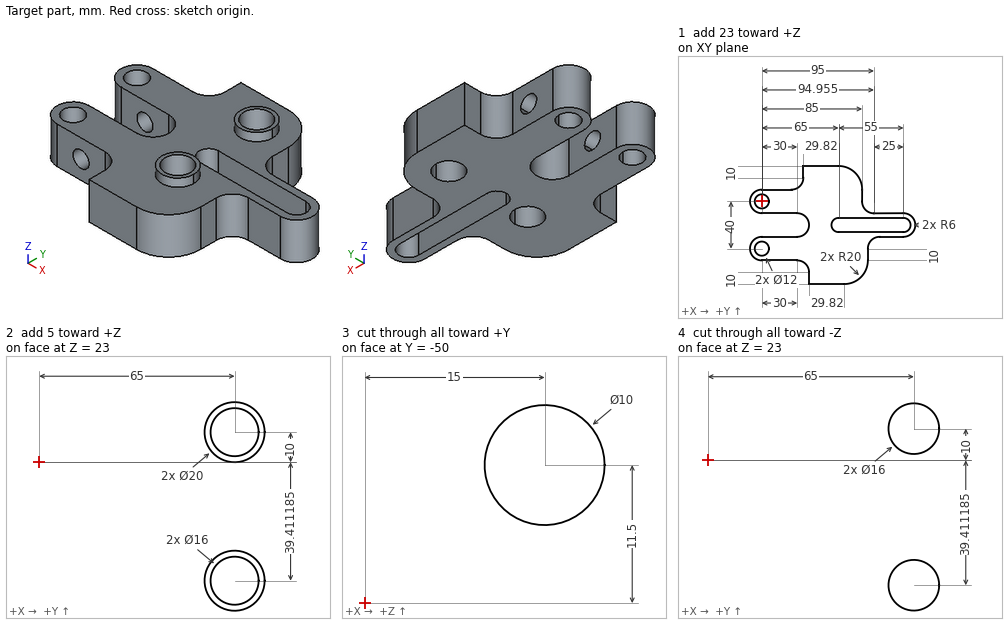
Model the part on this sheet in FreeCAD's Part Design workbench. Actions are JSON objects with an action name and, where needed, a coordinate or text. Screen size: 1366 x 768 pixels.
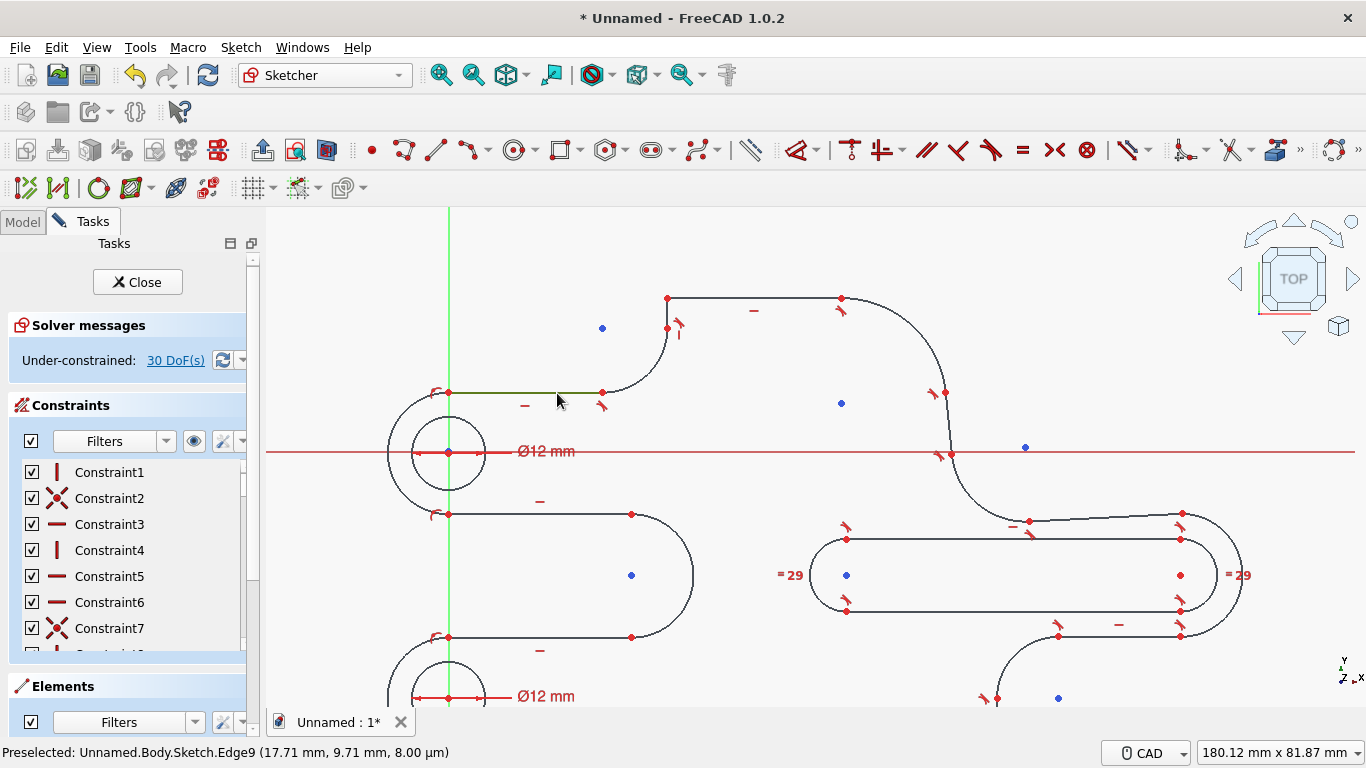
{"action": "left_click", "coordinate": [400, 418]}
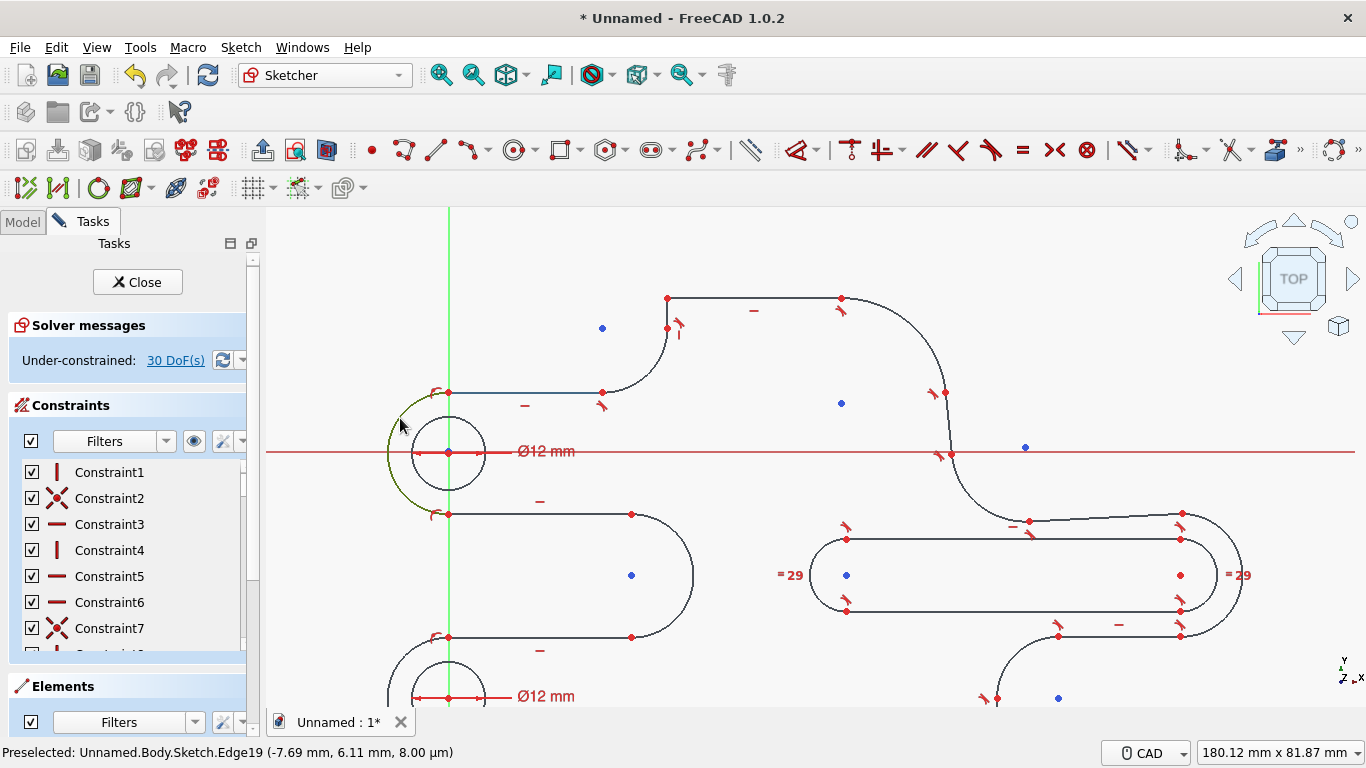
{"action": "key", "text": "t"}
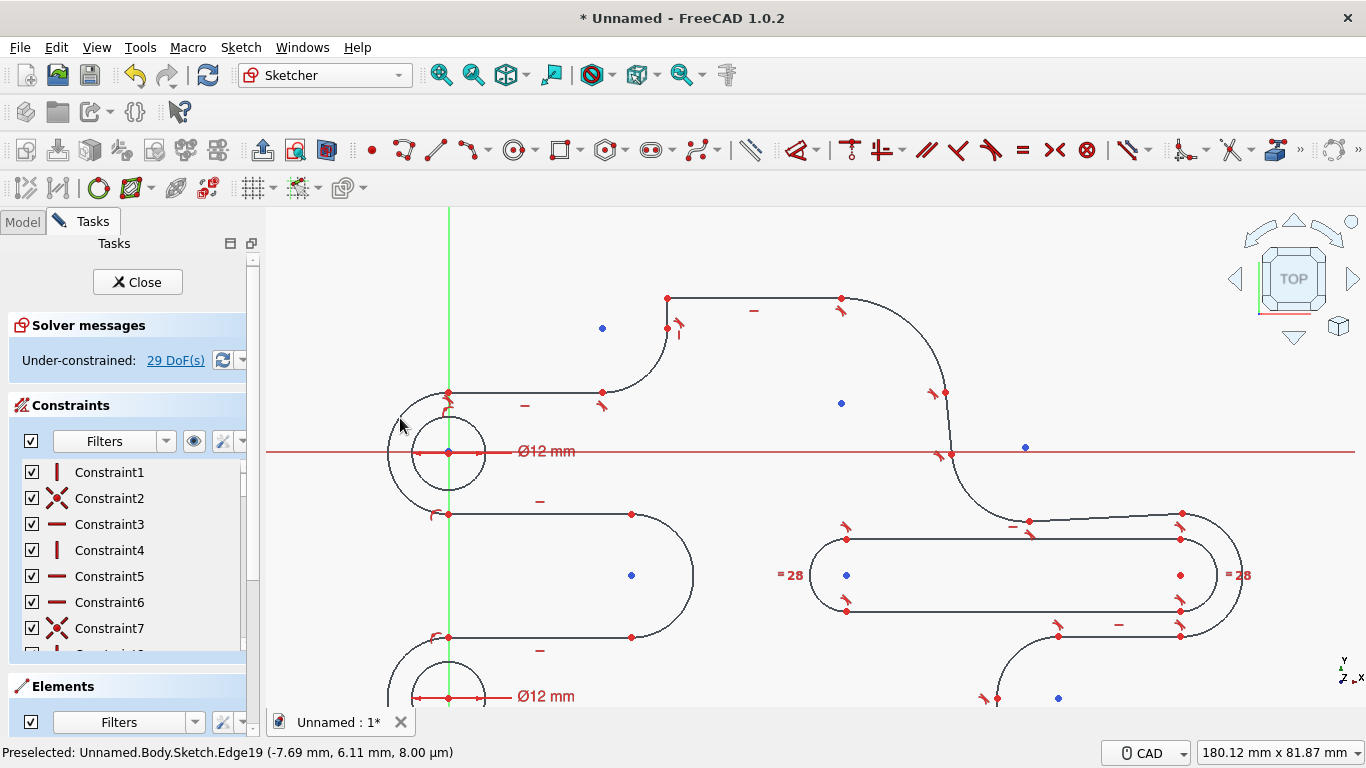
{"action": "left_click", "coordinate": [504, 514]}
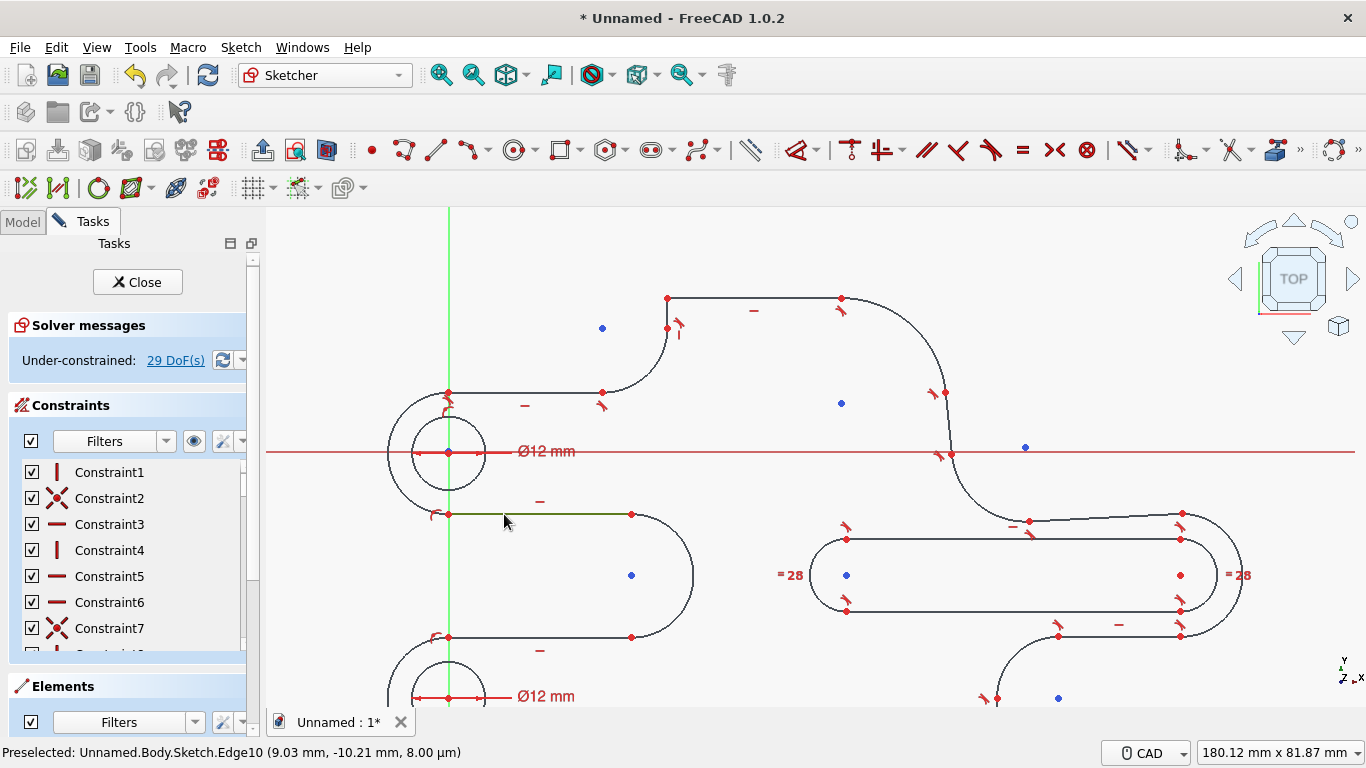
{"action": "left_click", "coordinate": [682, 612]}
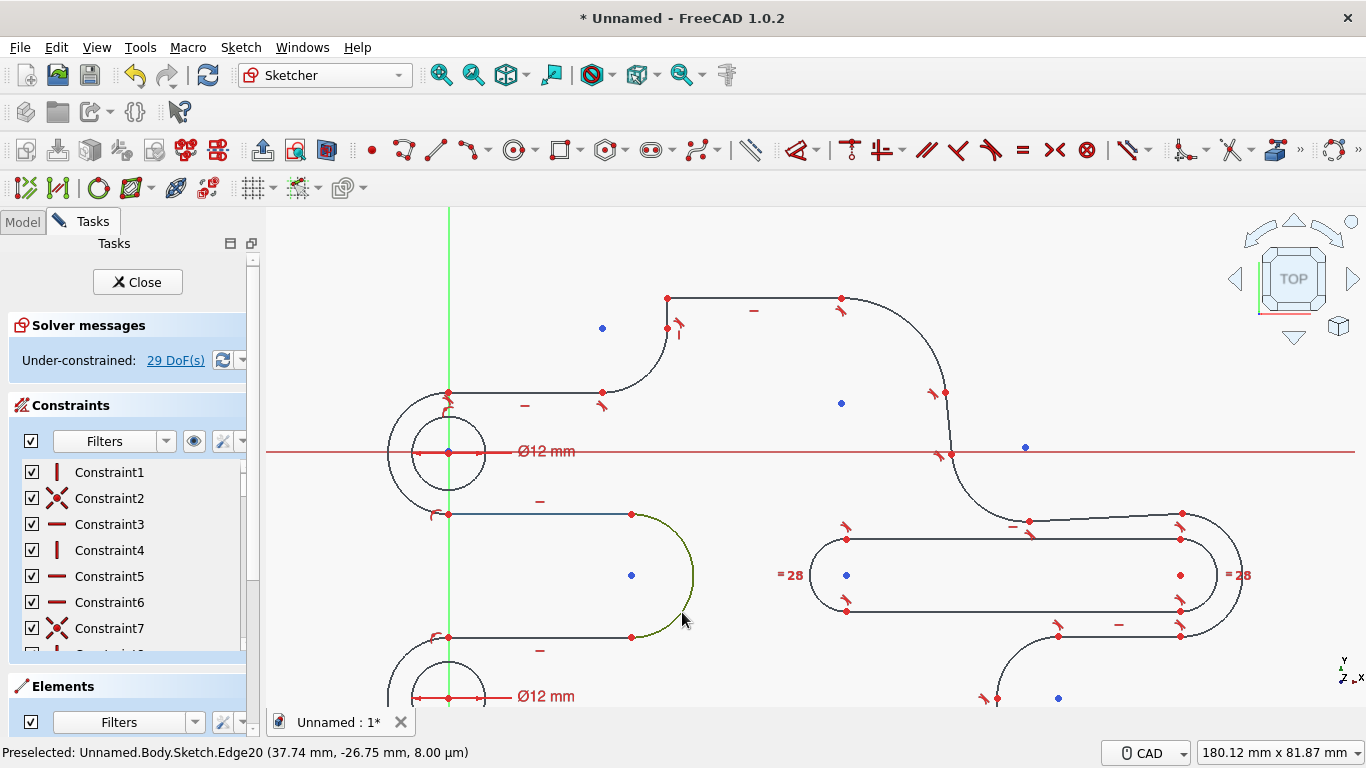
{"action": "left_click", "coordinate": [992, 150]}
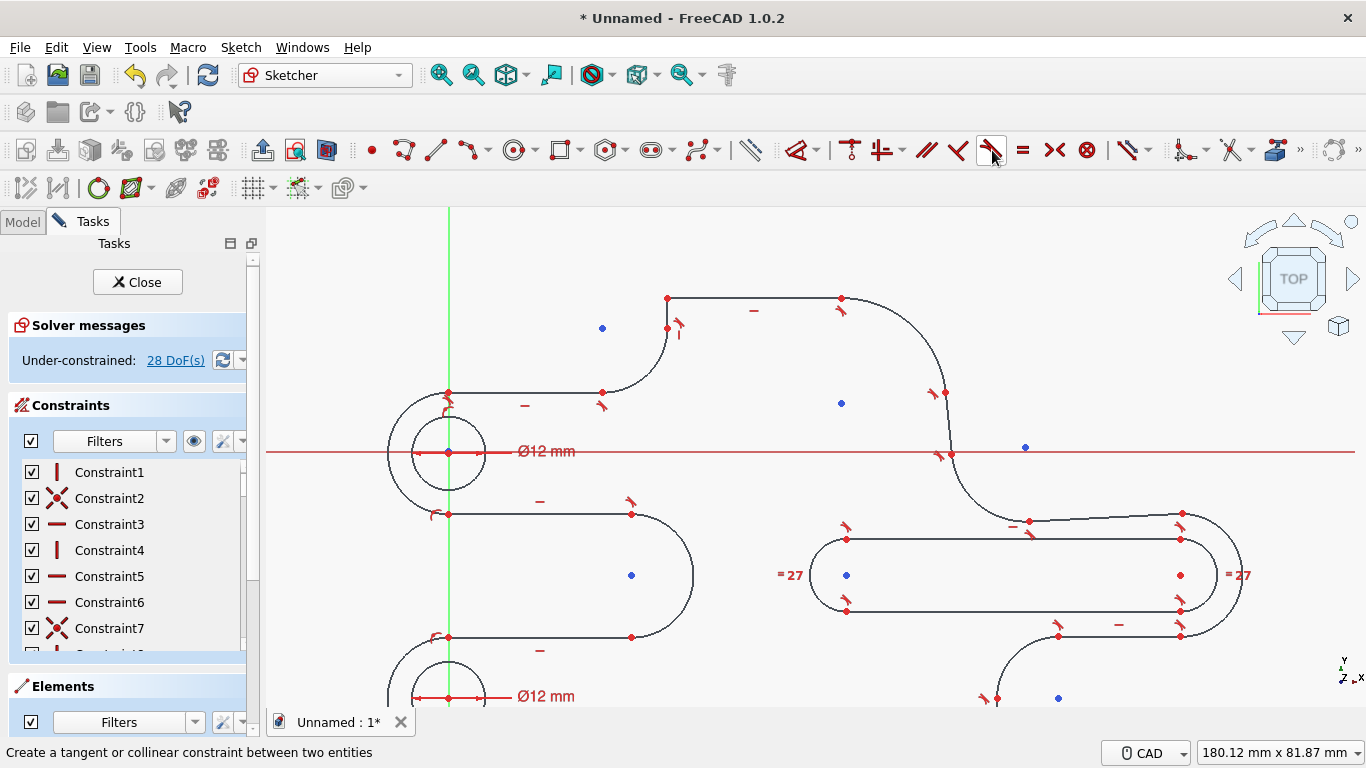
{"action": "left_click", "coordinate": [577, 638]}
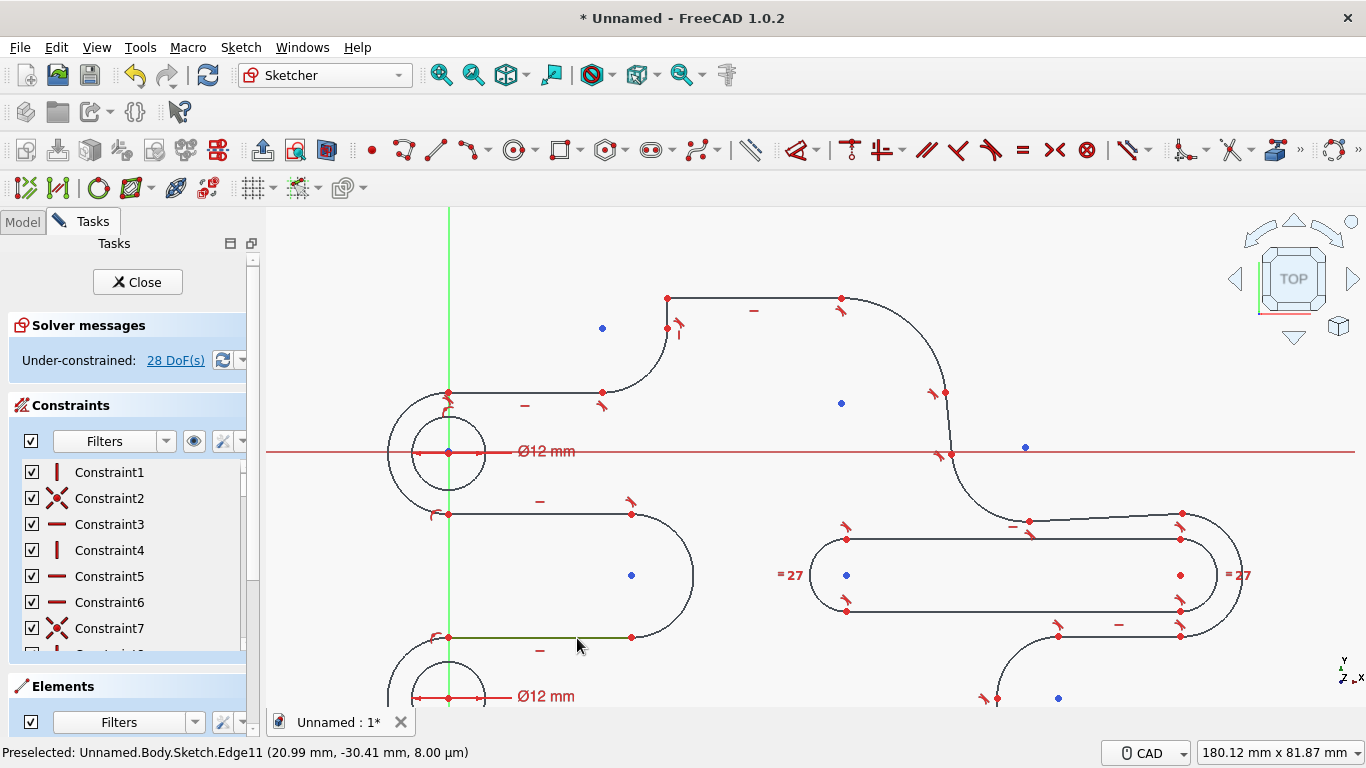
{"action": "left_click", "coordinate": [682, 612]}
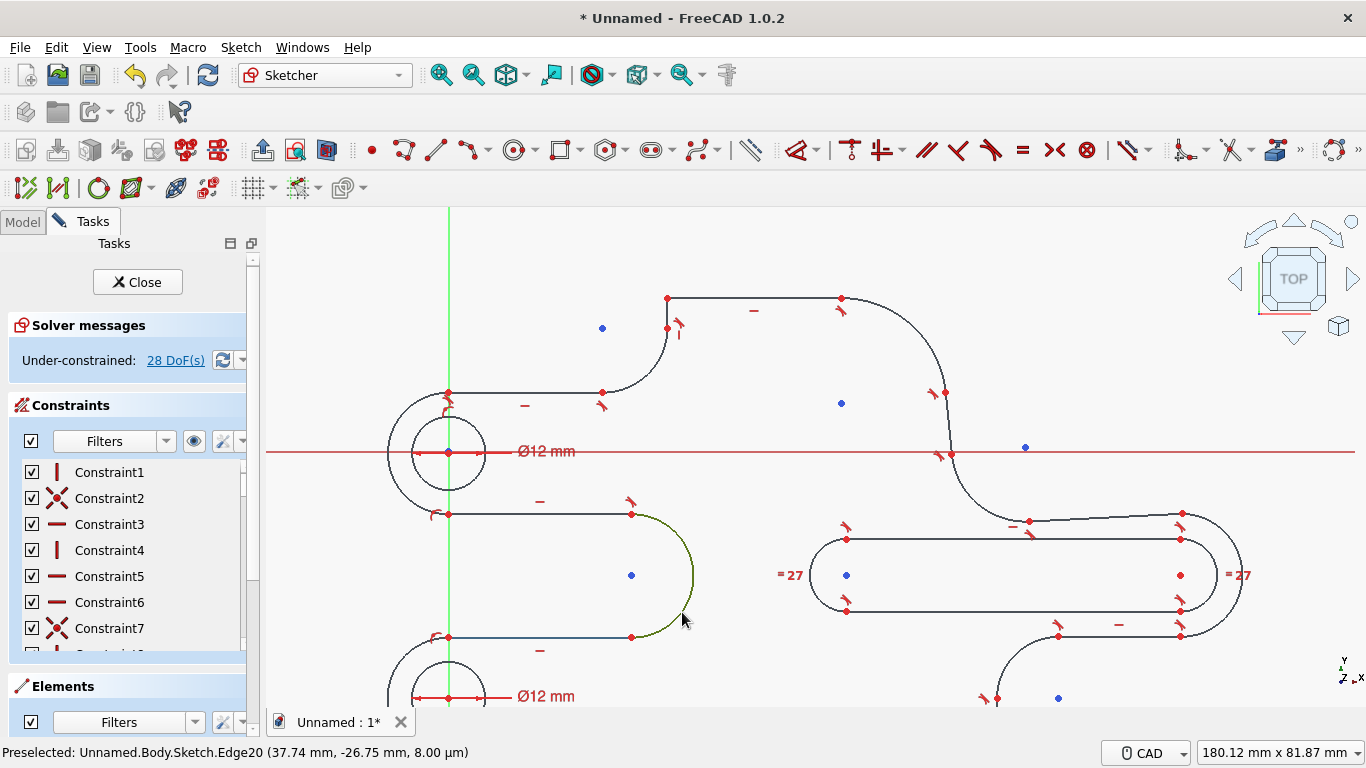
{"action": "key", "text": "t"}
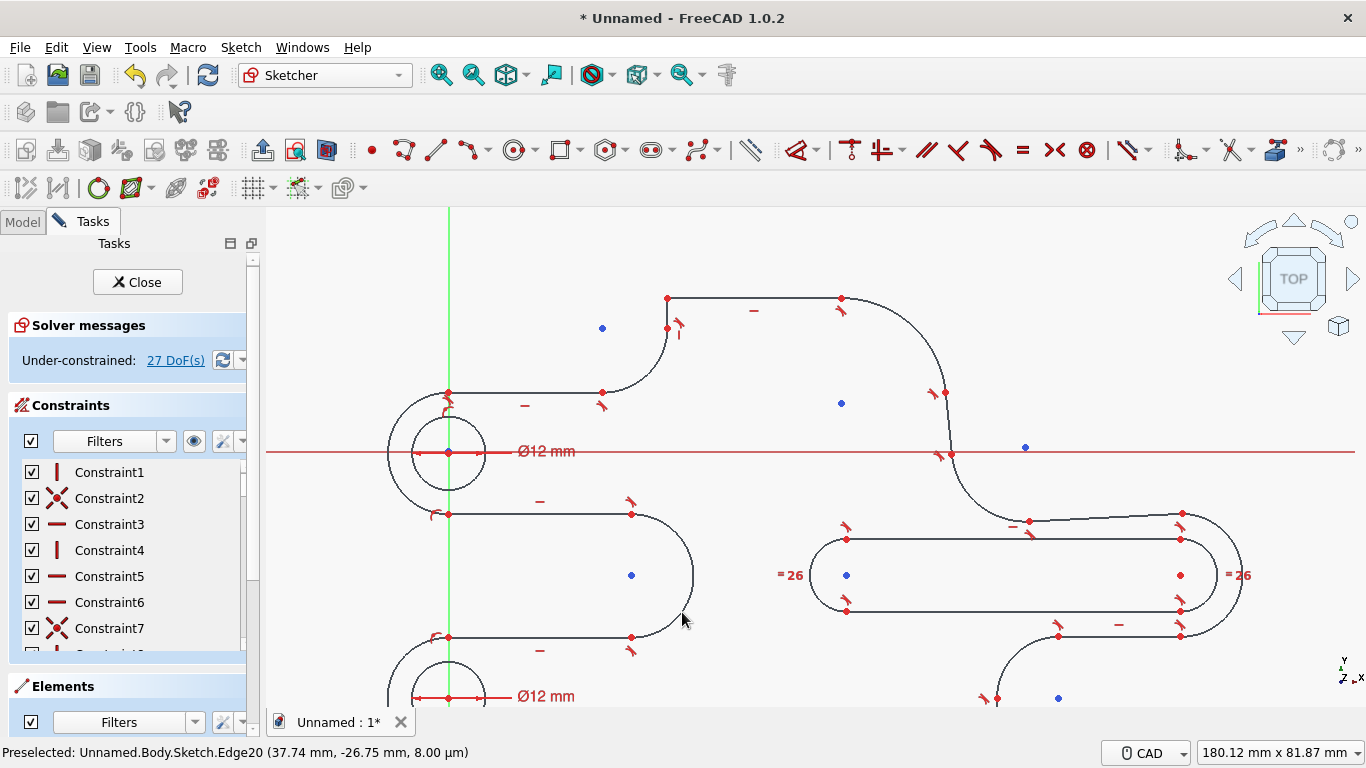
{"action": "left_click", "coordinate": [577, 638]}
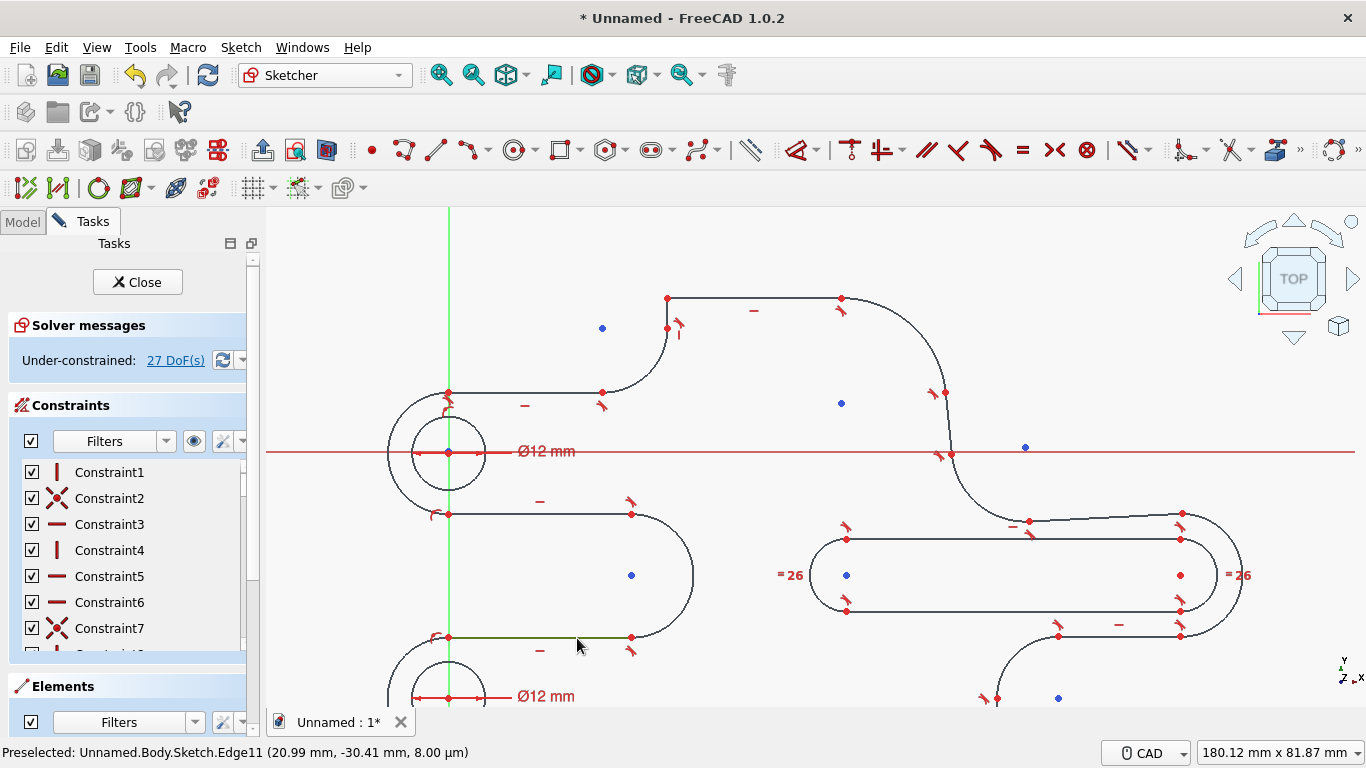
{"action": "left_click", "coordinate": [399, 663]}